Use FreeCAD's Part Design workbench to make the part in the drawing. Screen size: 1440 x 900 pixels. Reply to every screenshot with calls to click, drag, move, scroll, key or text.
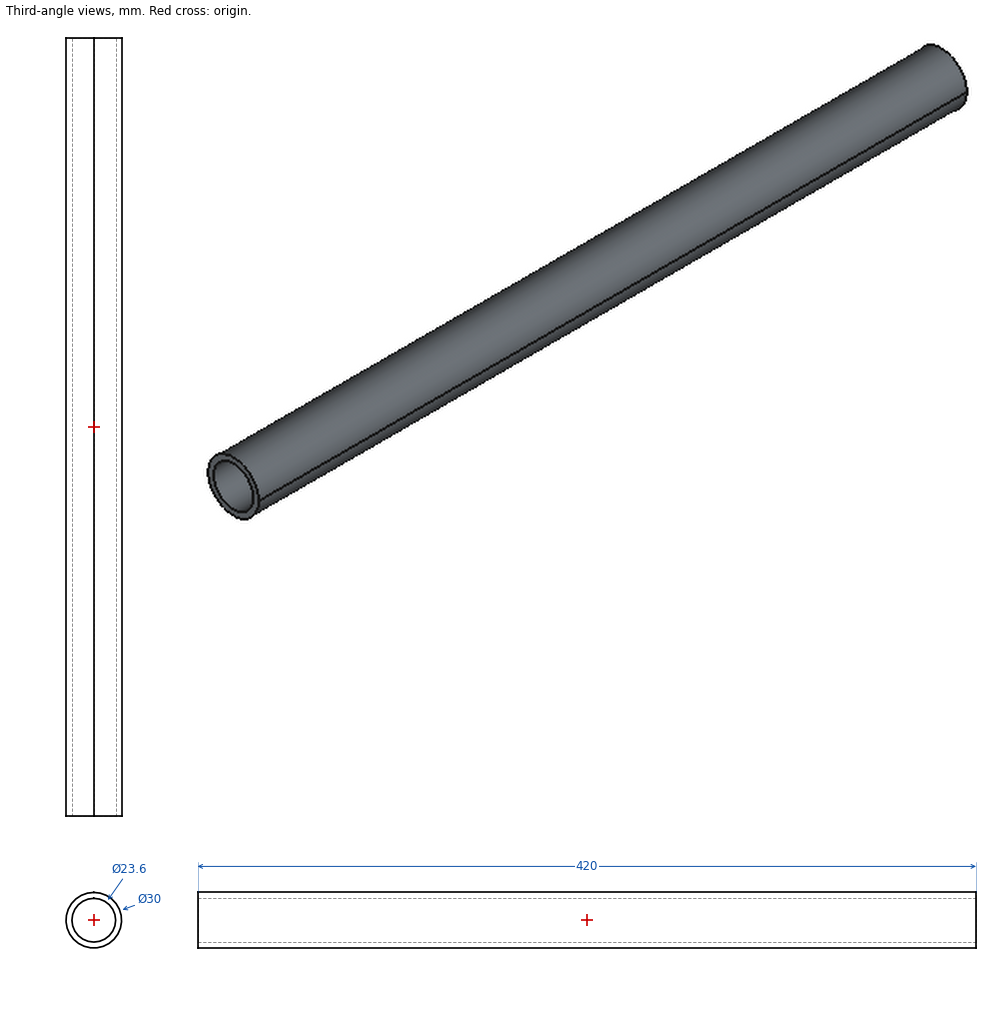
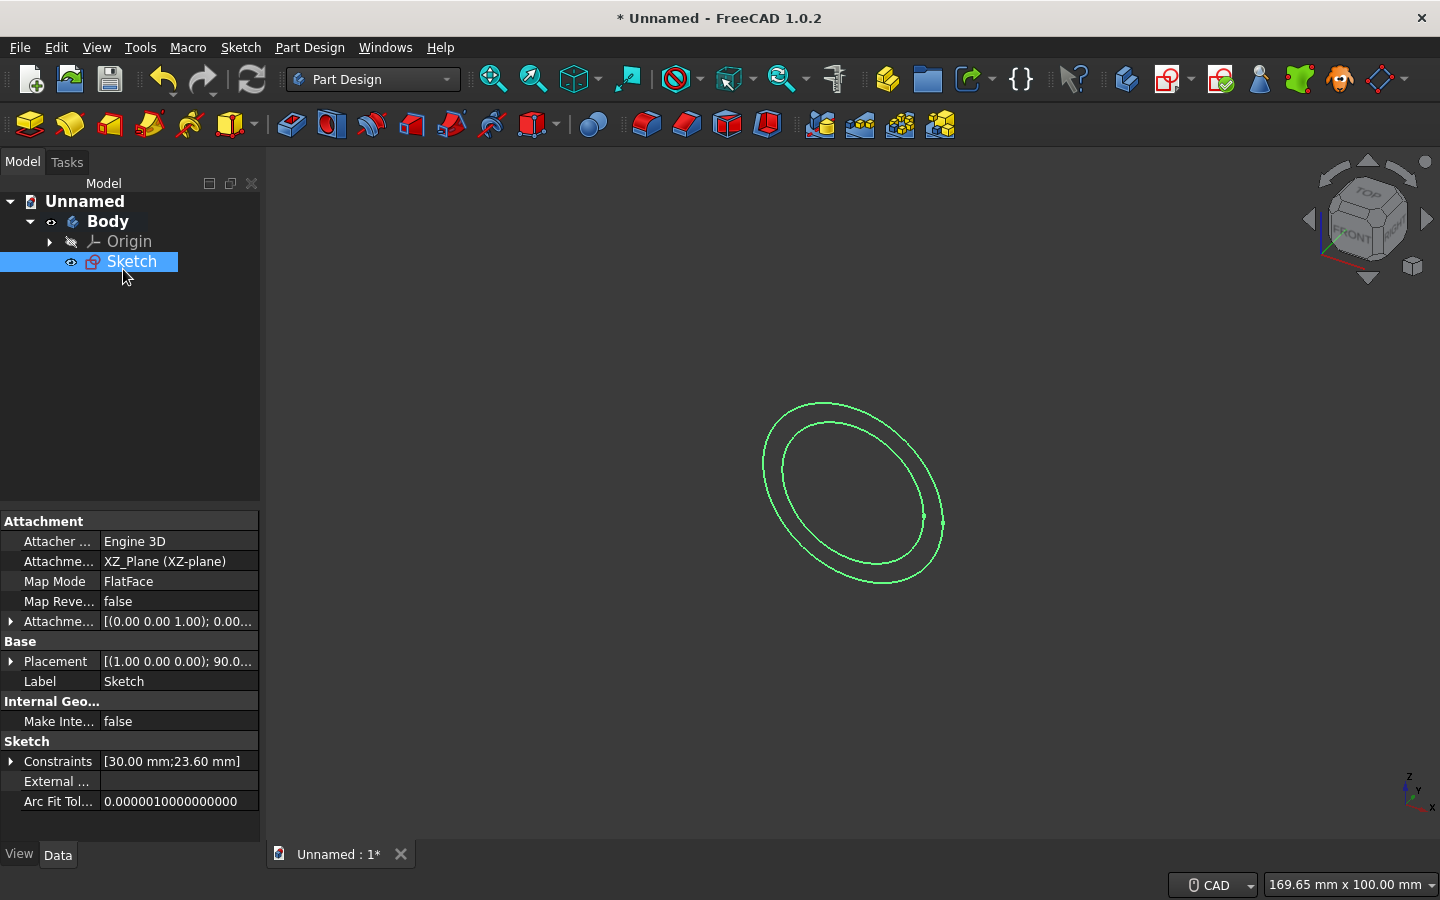
click(30, 124)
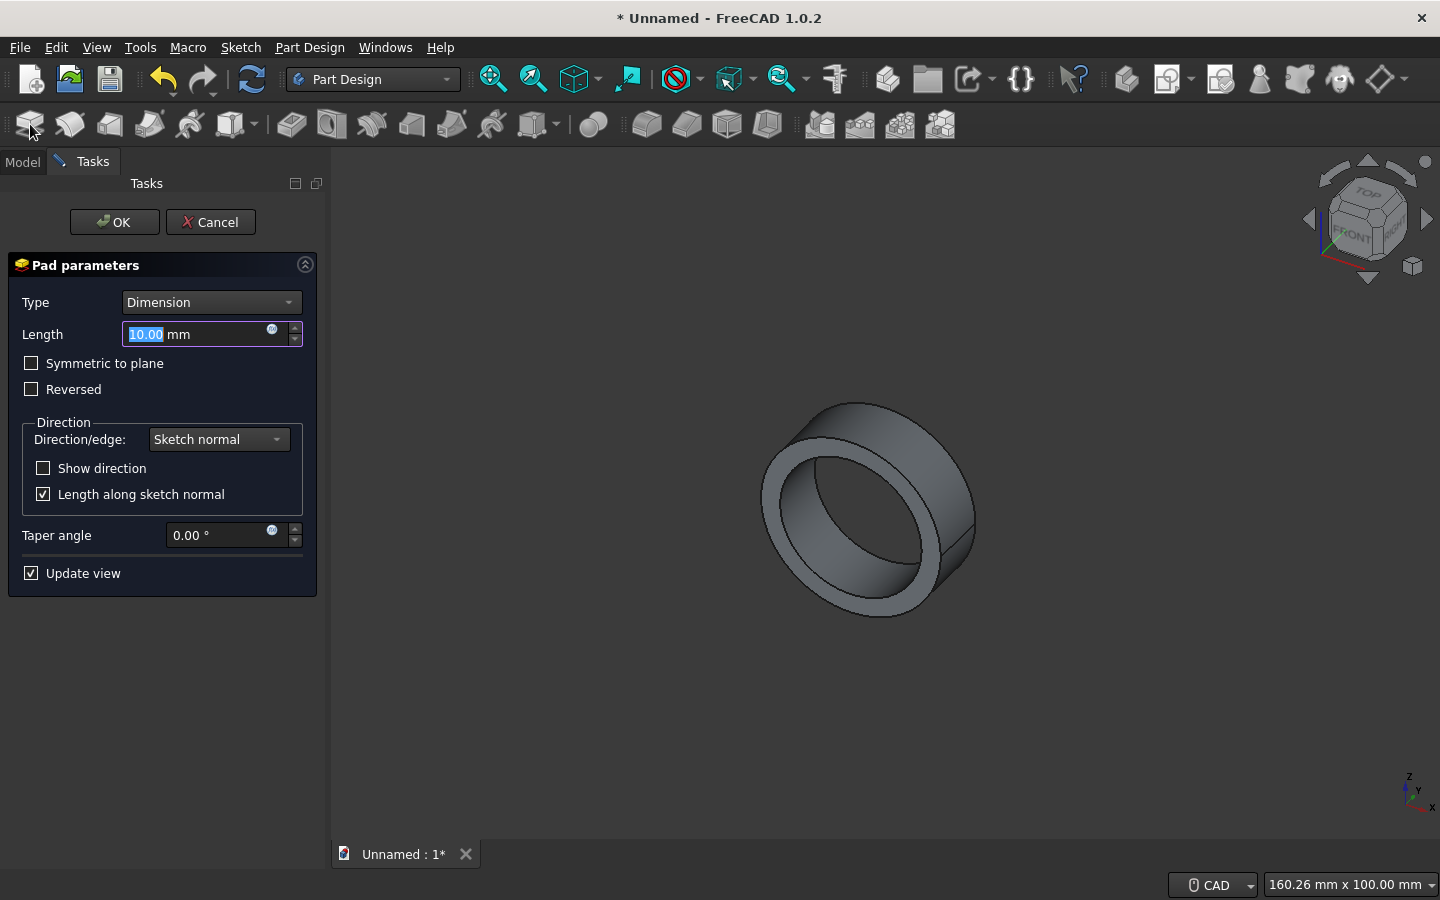
text(420)
key(Tab)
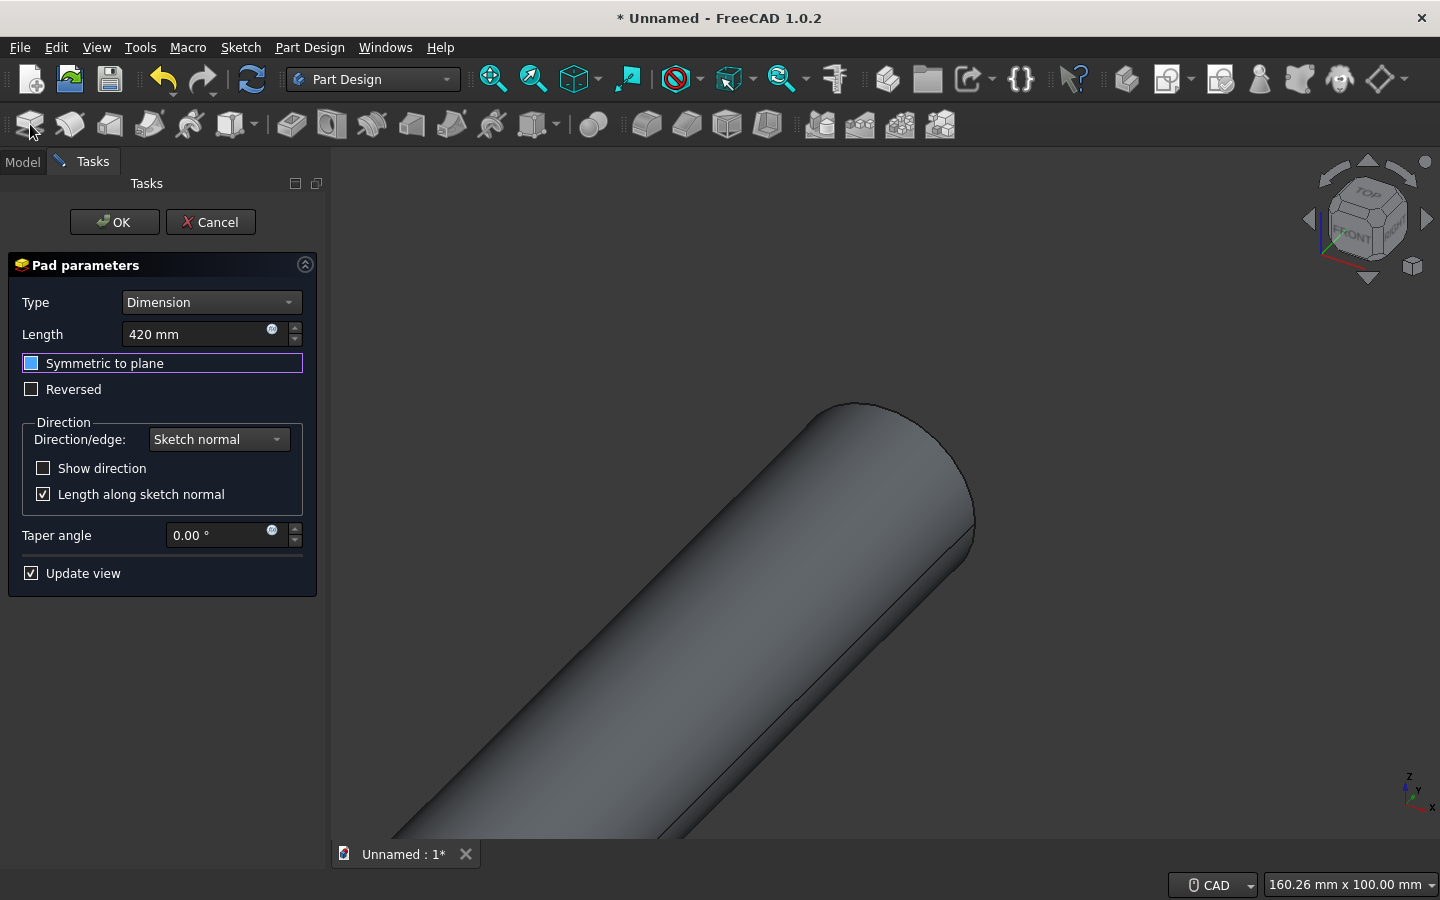
click(30, 363)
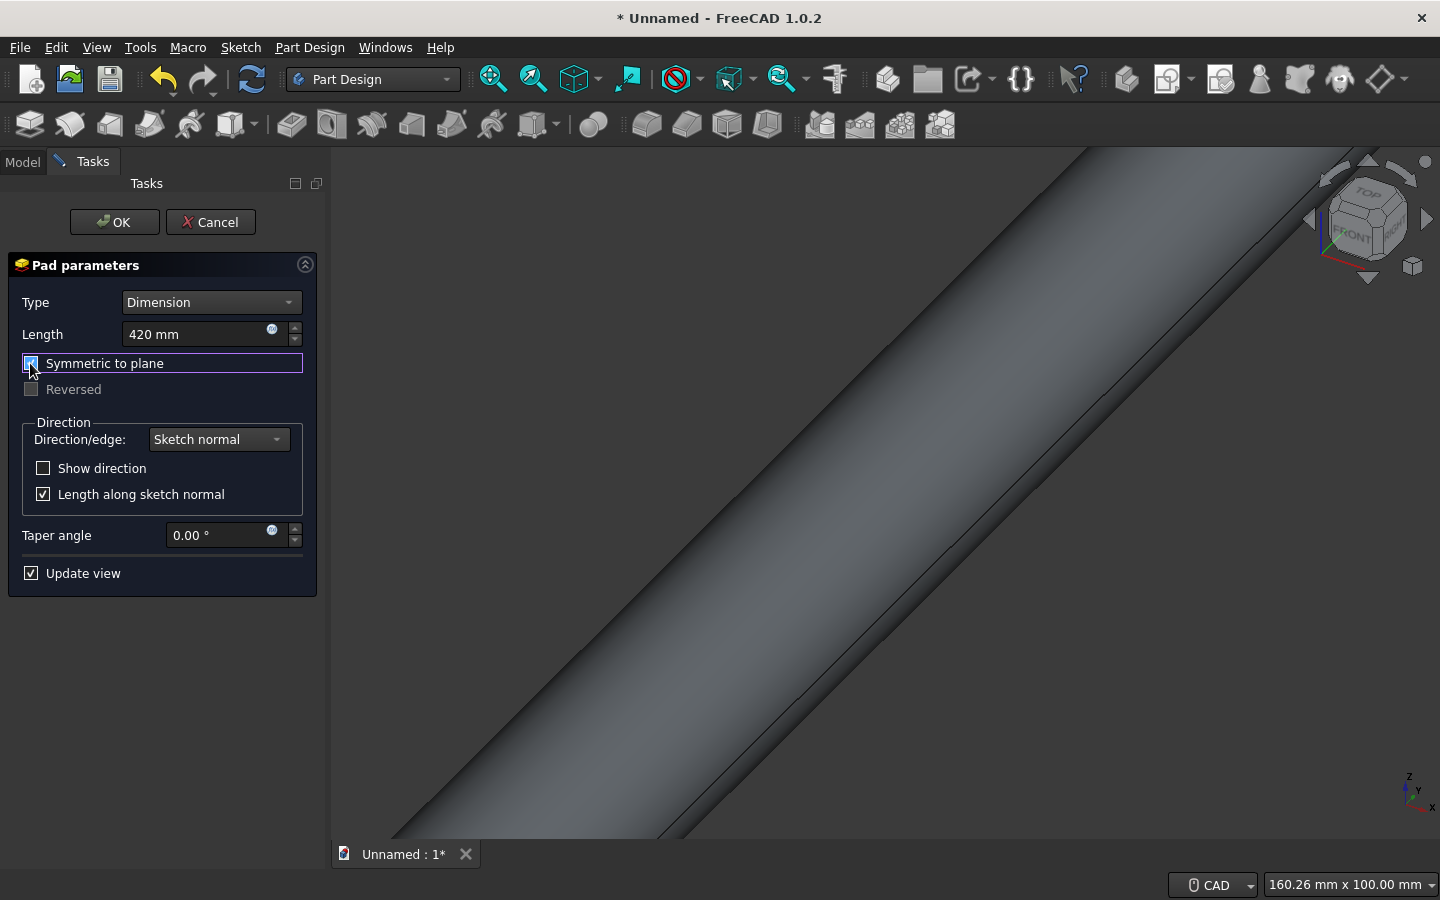
click(115, 222)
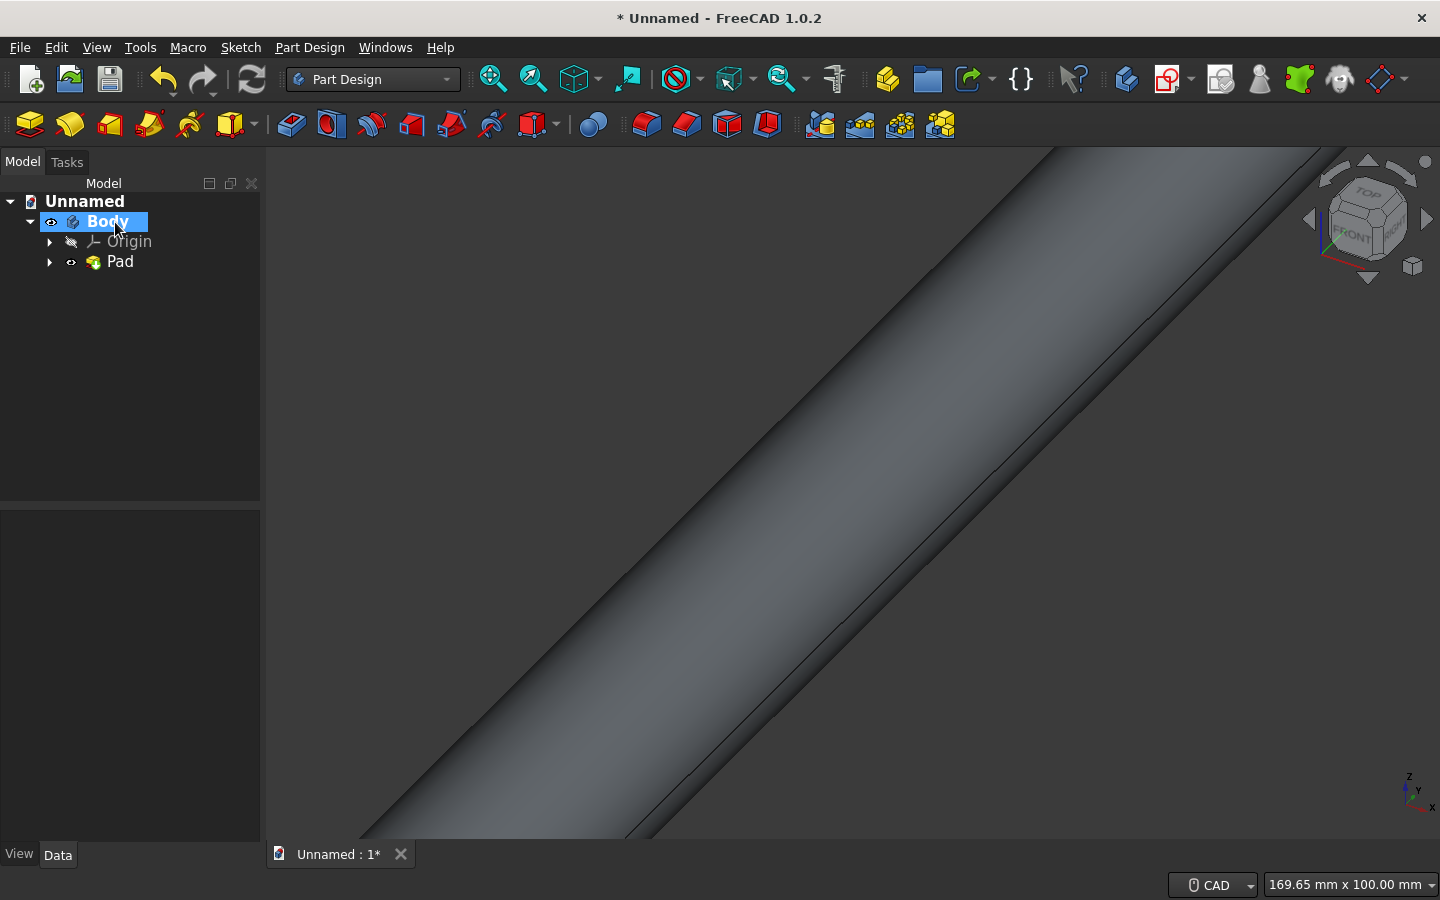
key(0)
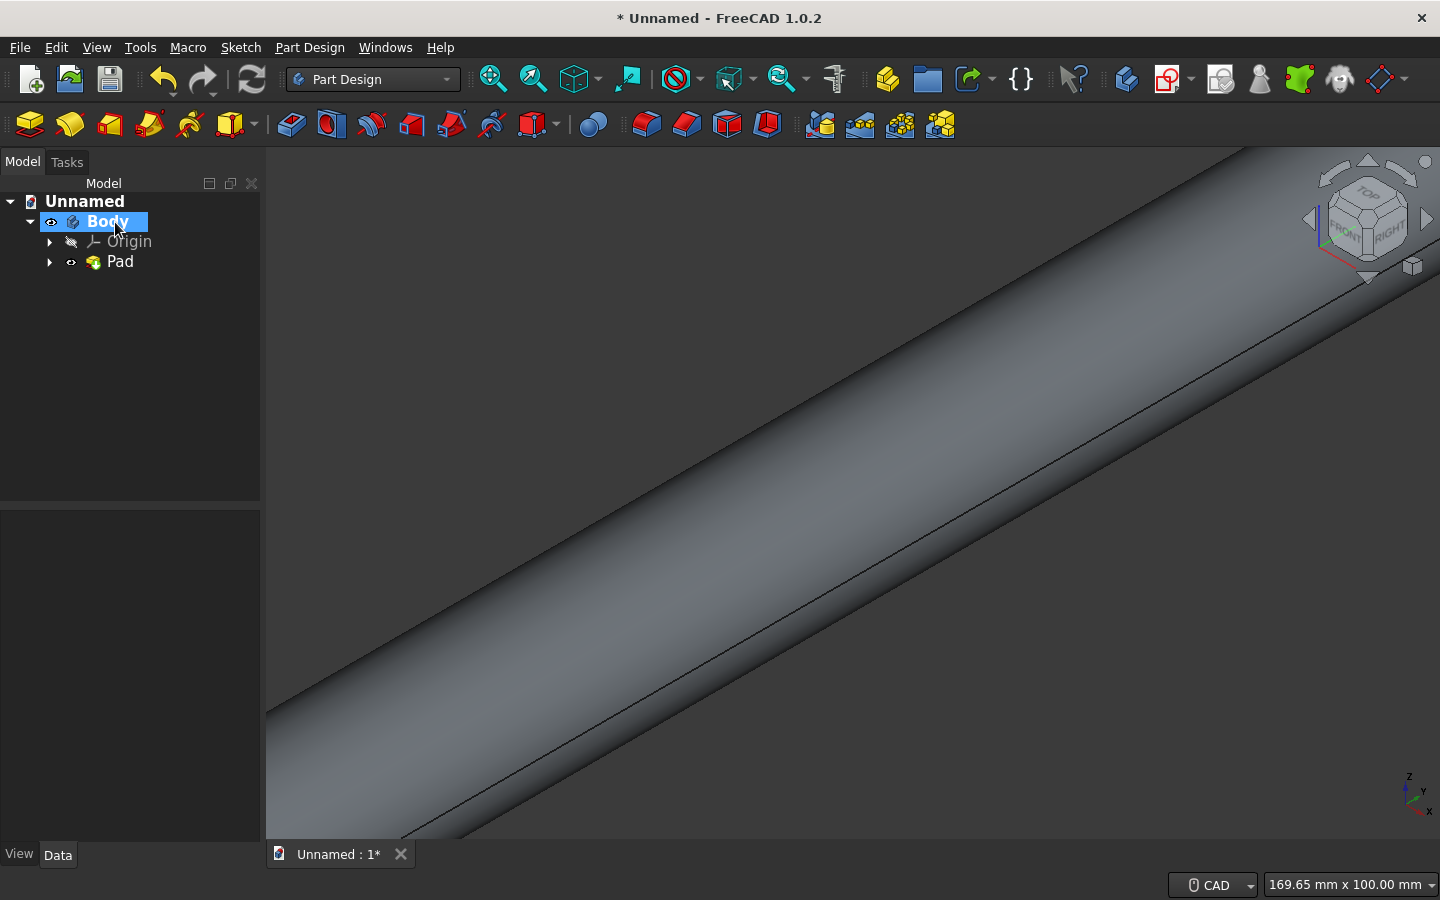
click(494, 80)